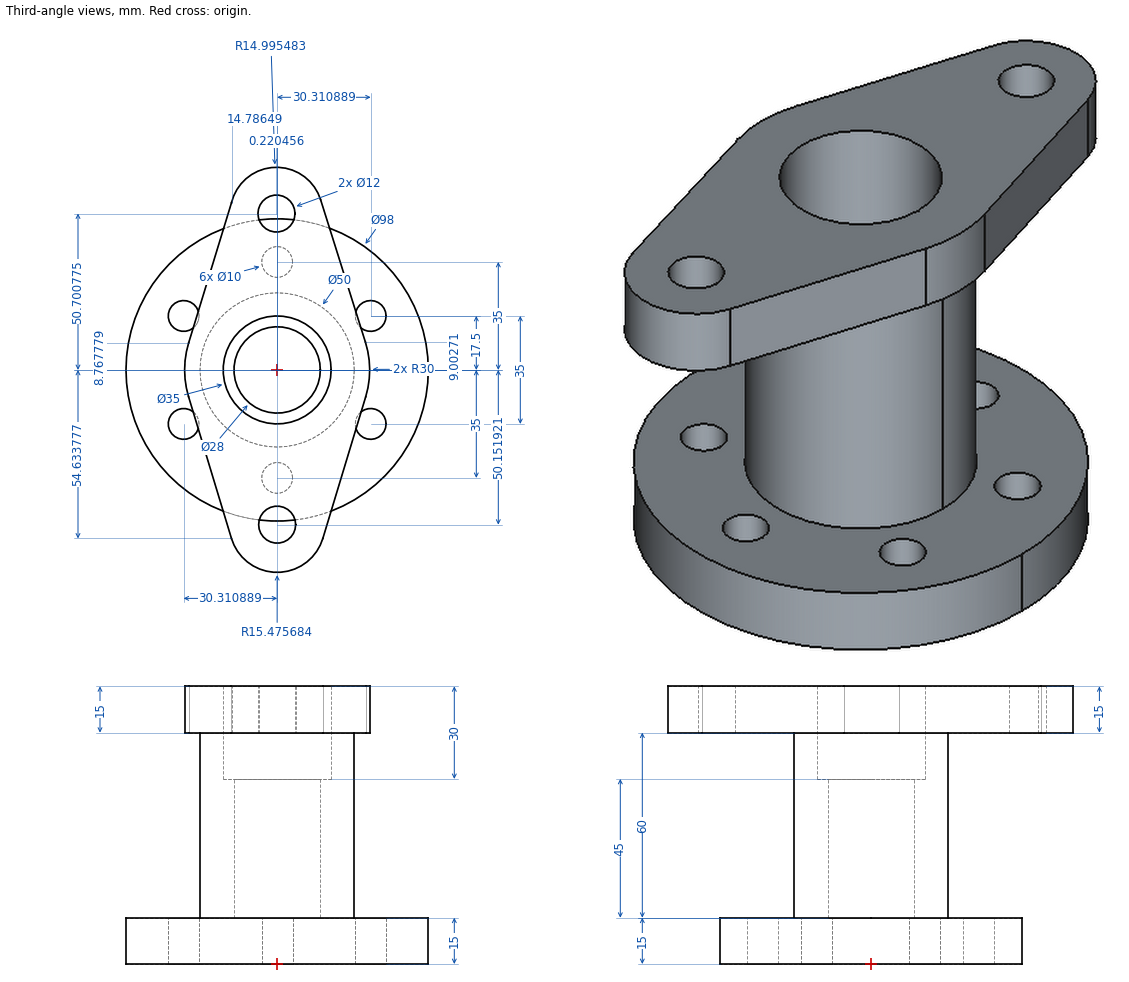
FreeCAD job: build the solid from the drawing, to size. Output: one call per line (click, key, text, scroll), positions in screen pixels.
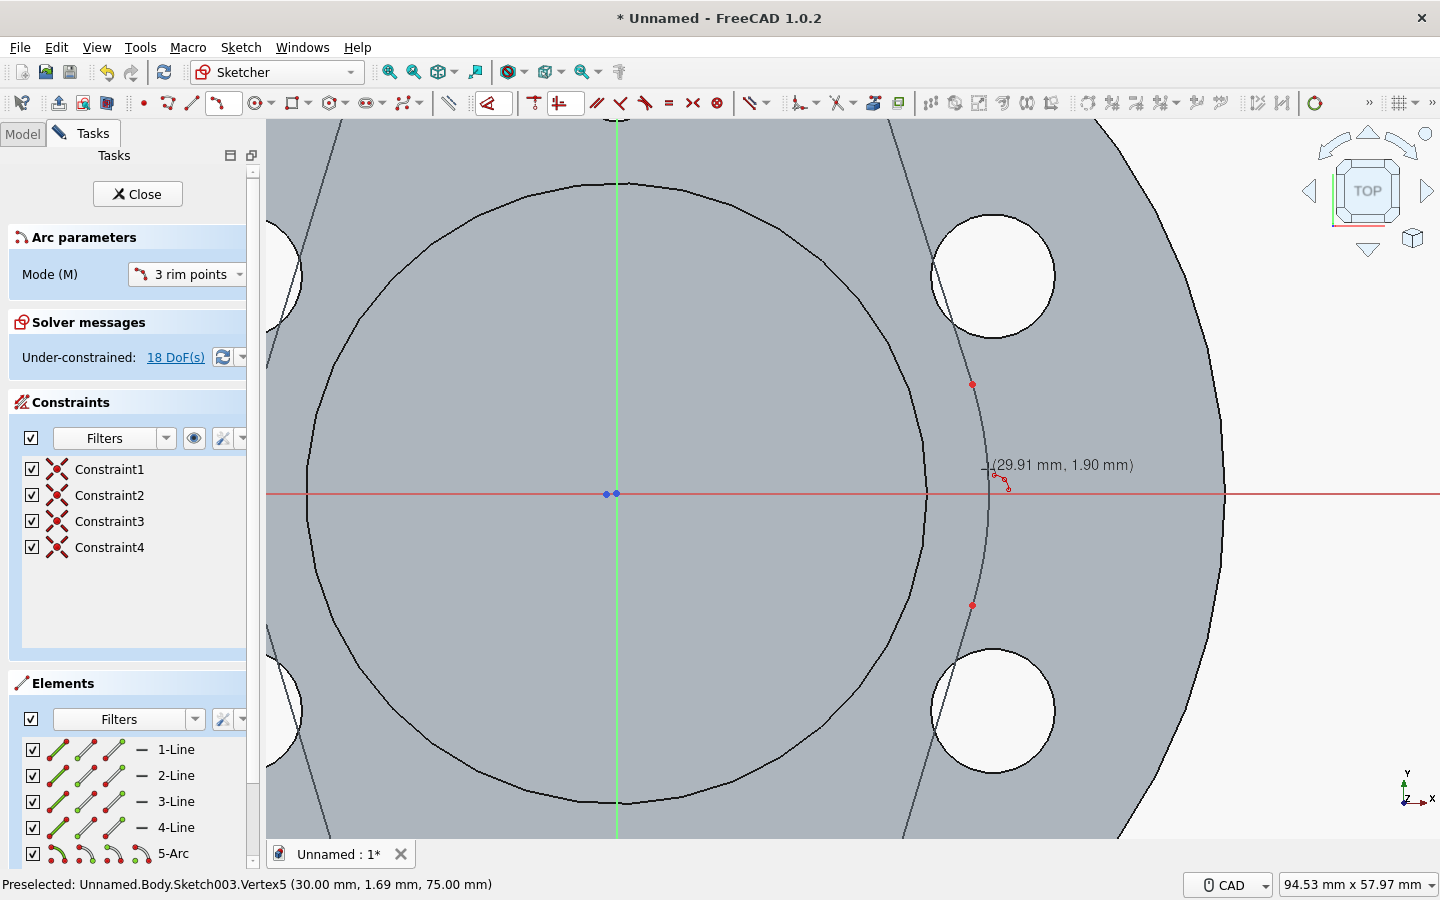
scroll(857, 473, down, 6)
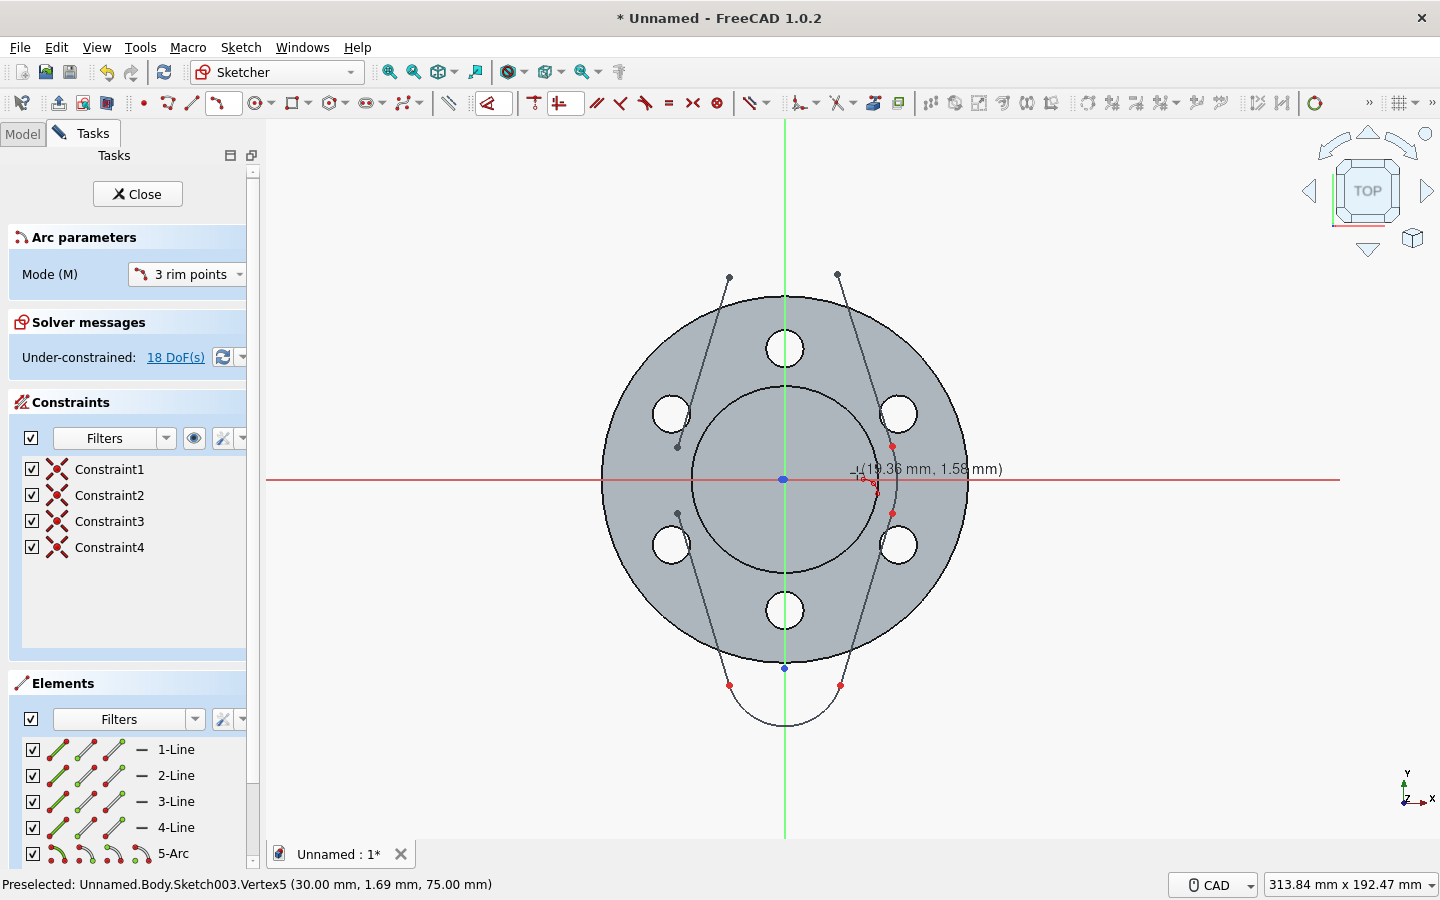
click(837, 274)
click(729, 277)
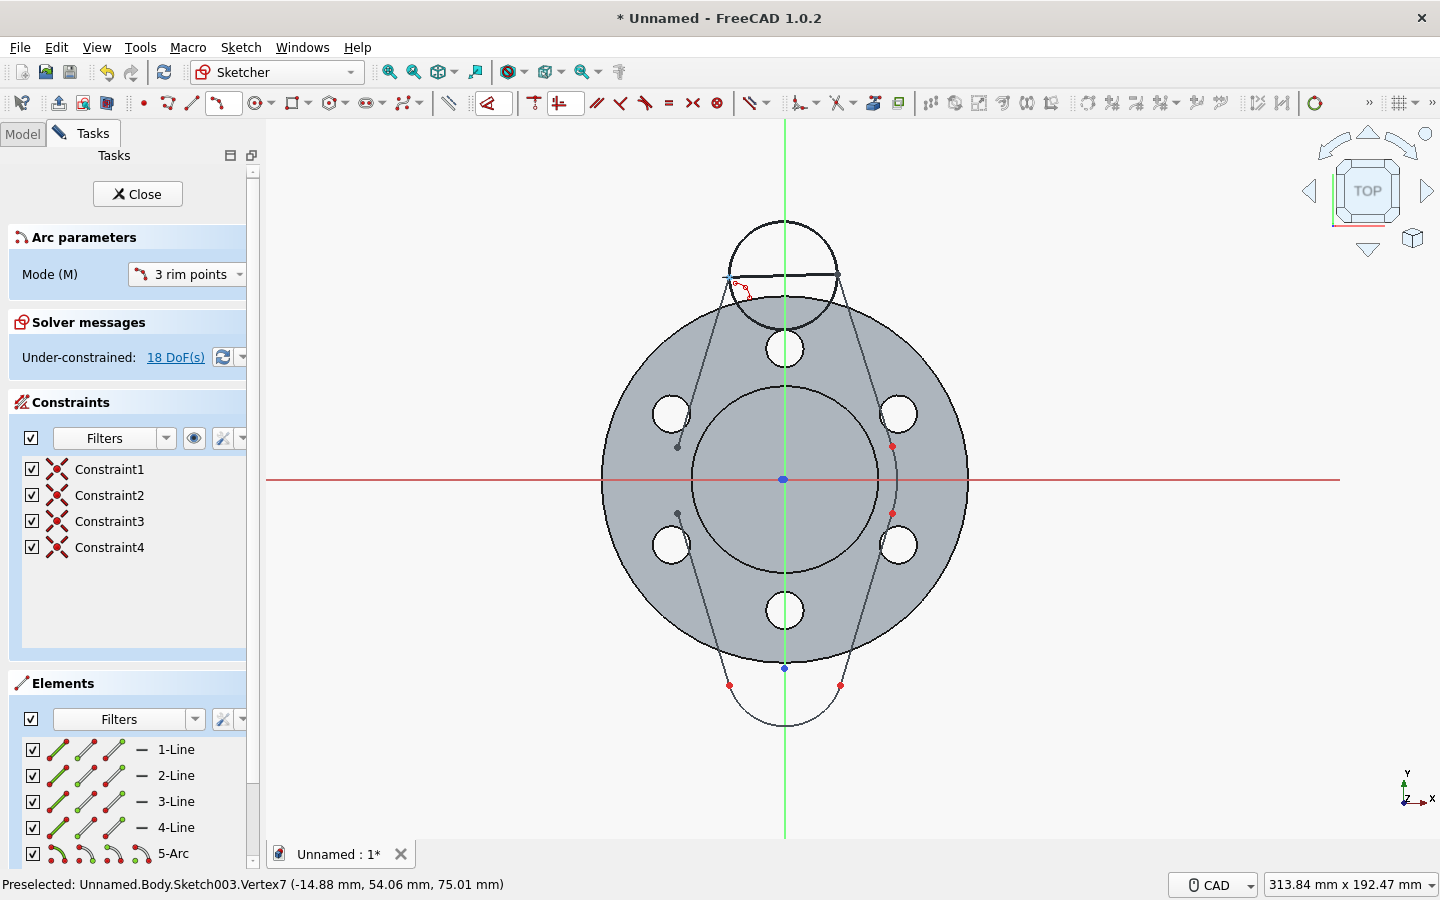
scroll(797, 235, up, 2)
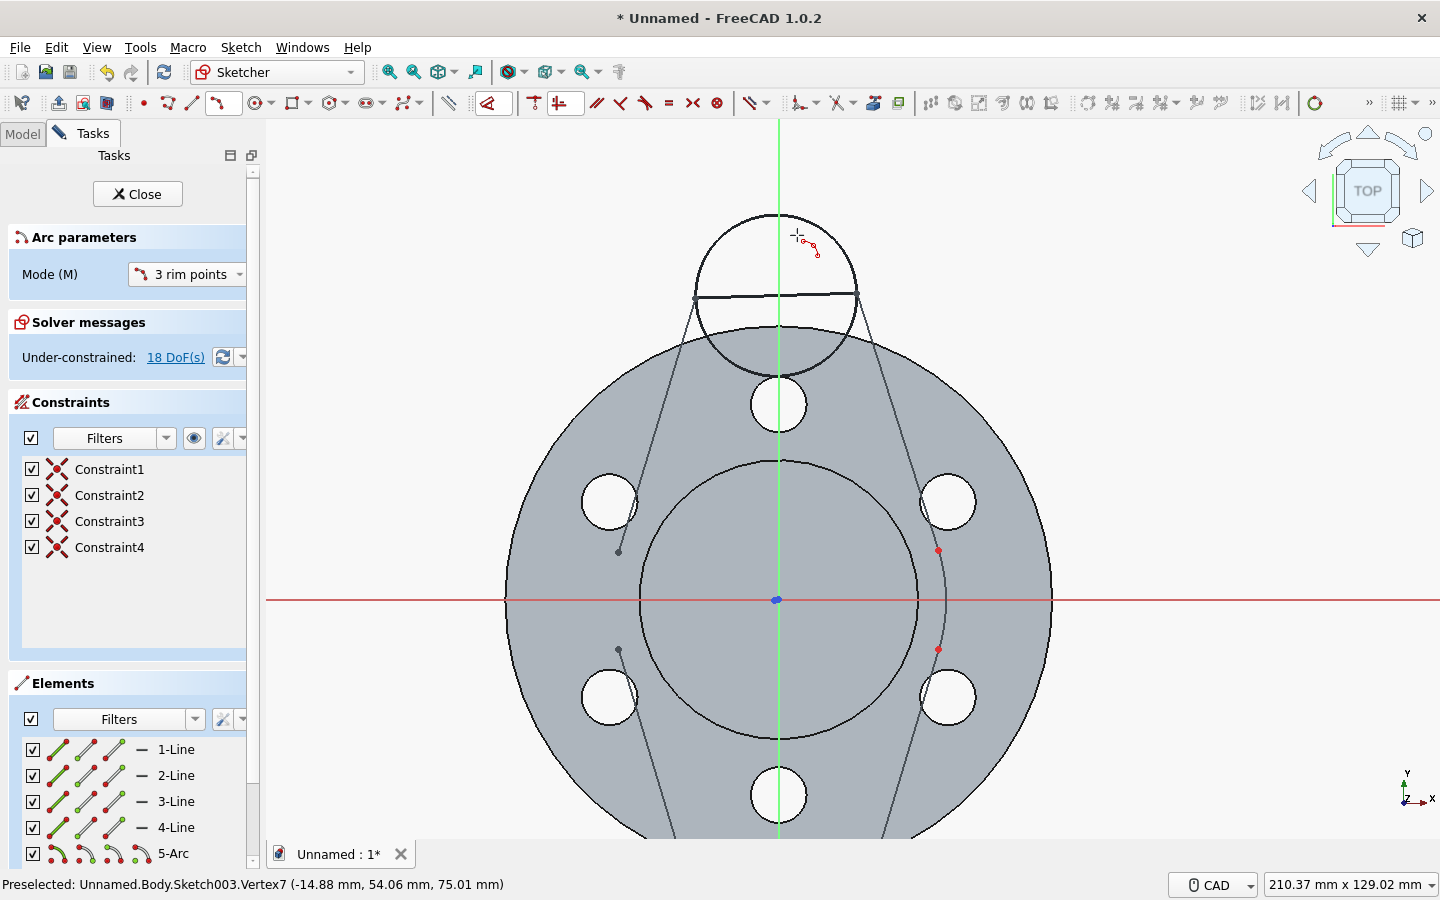
click(796, 235)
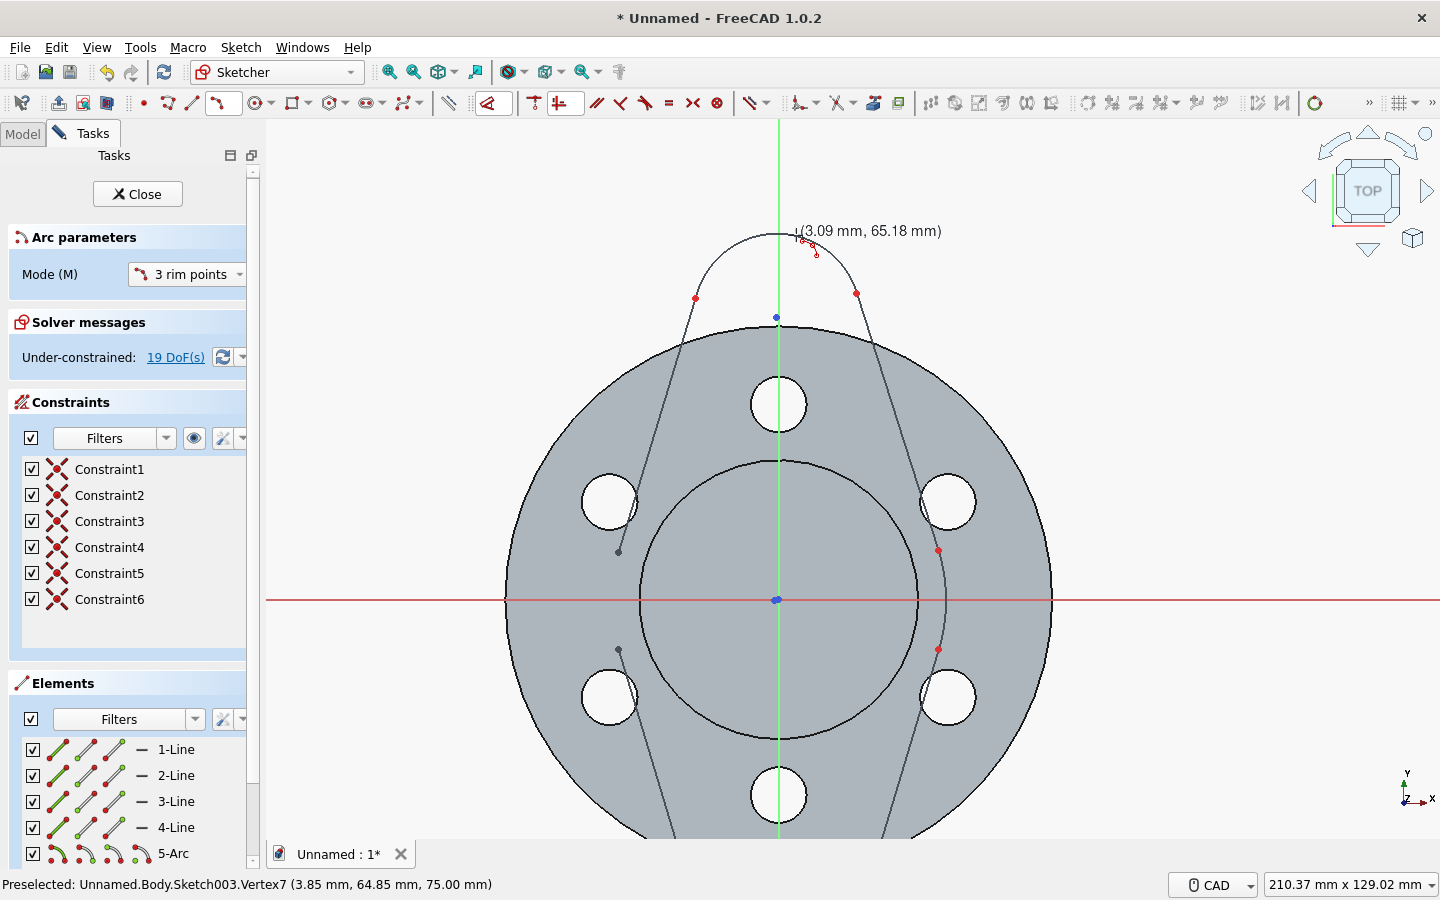
click(619, 552)
click(619, 650)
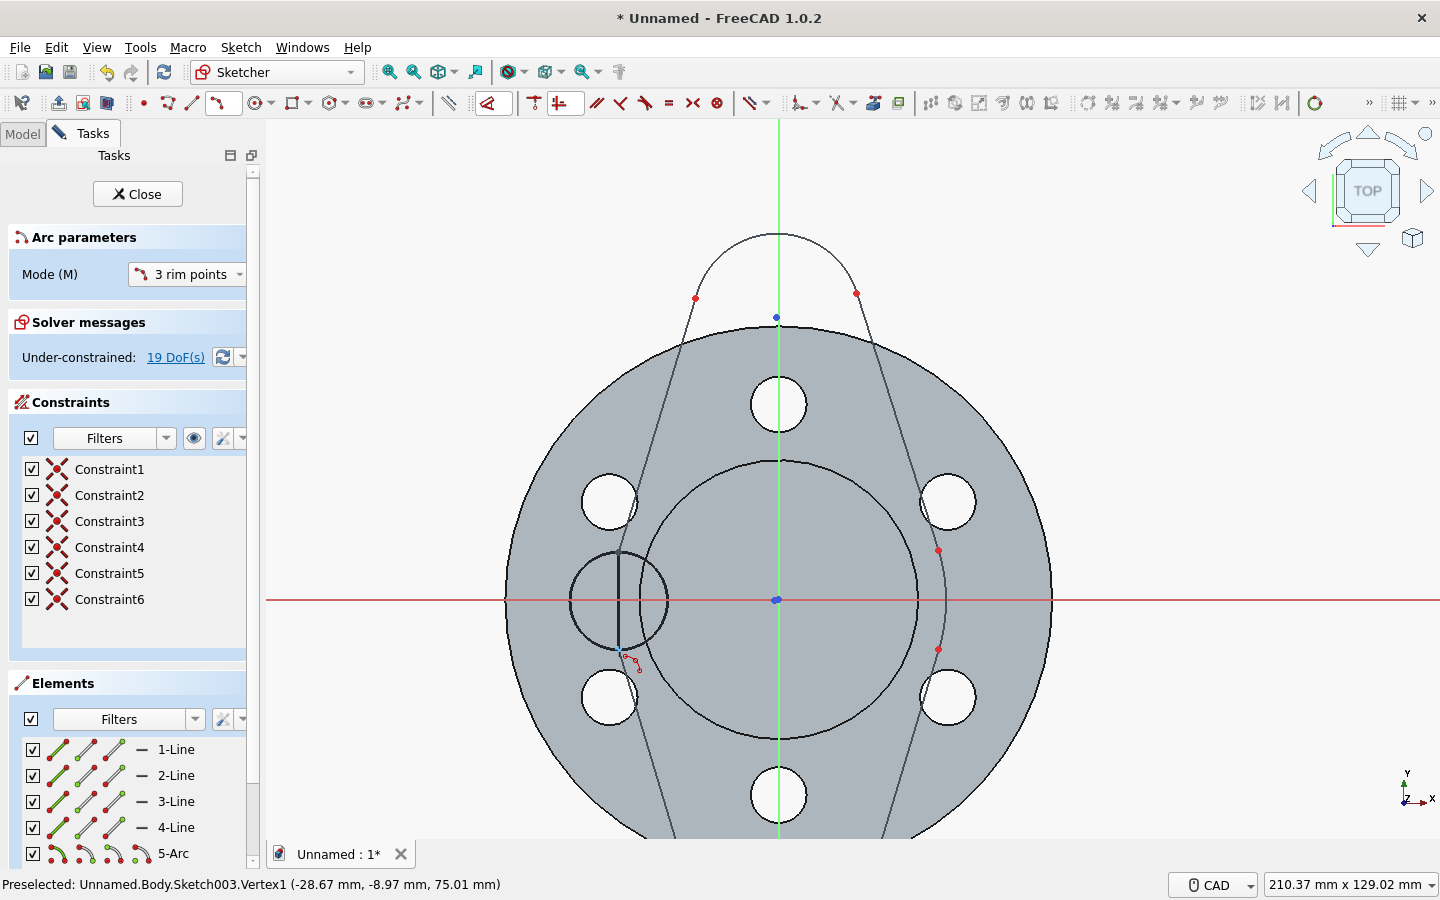
scroll(612, 609, up, 5)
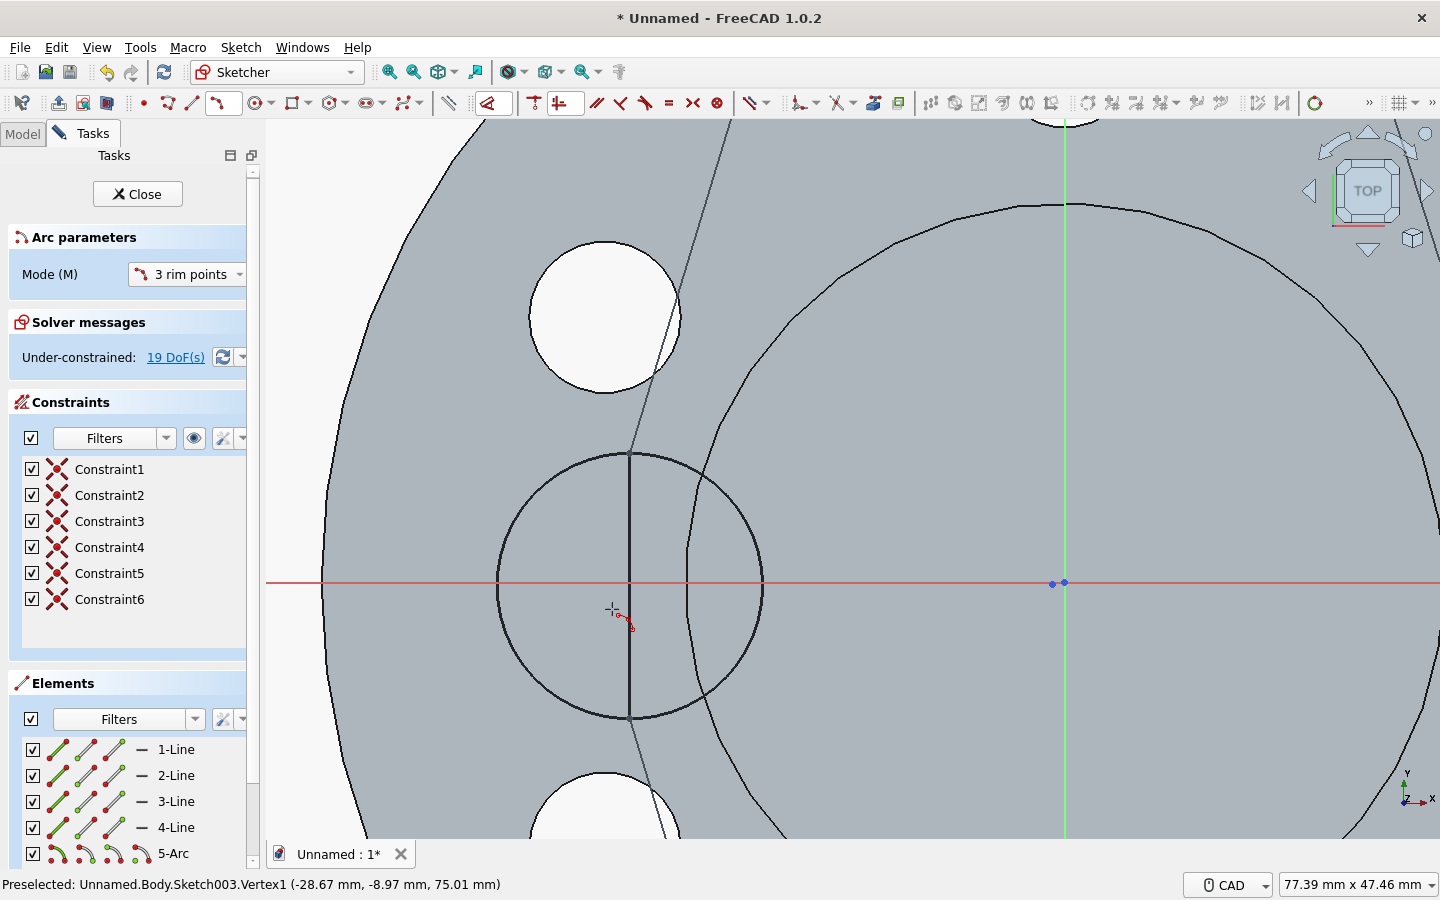
click(610, 609)
key(Escape)